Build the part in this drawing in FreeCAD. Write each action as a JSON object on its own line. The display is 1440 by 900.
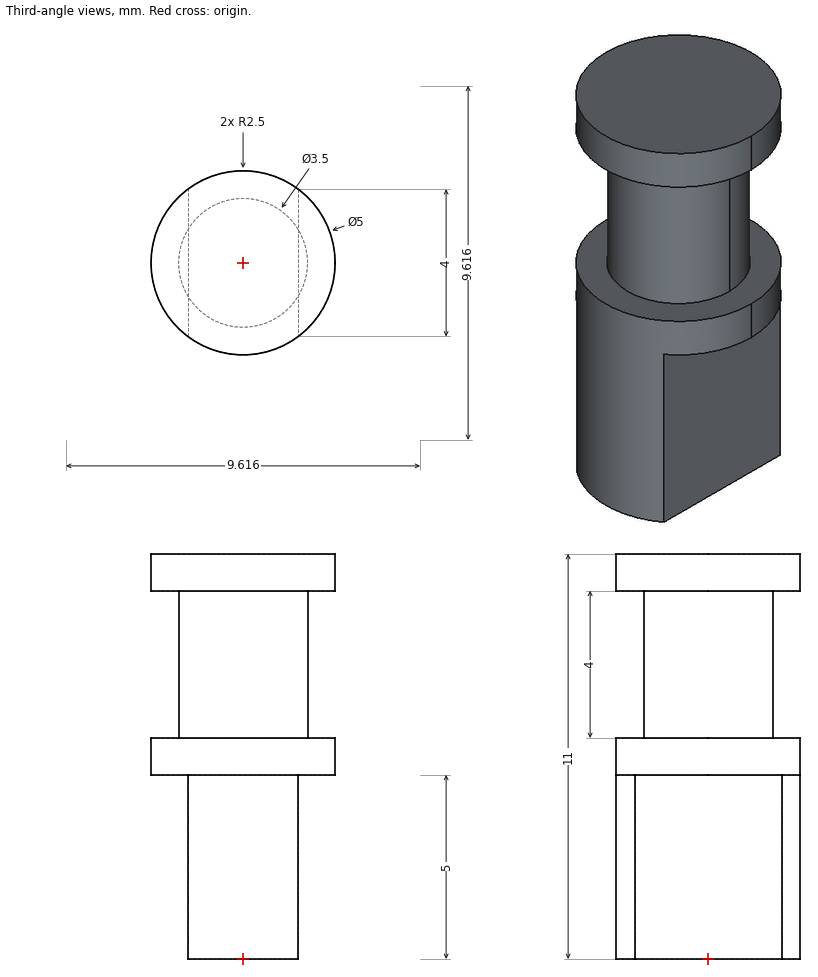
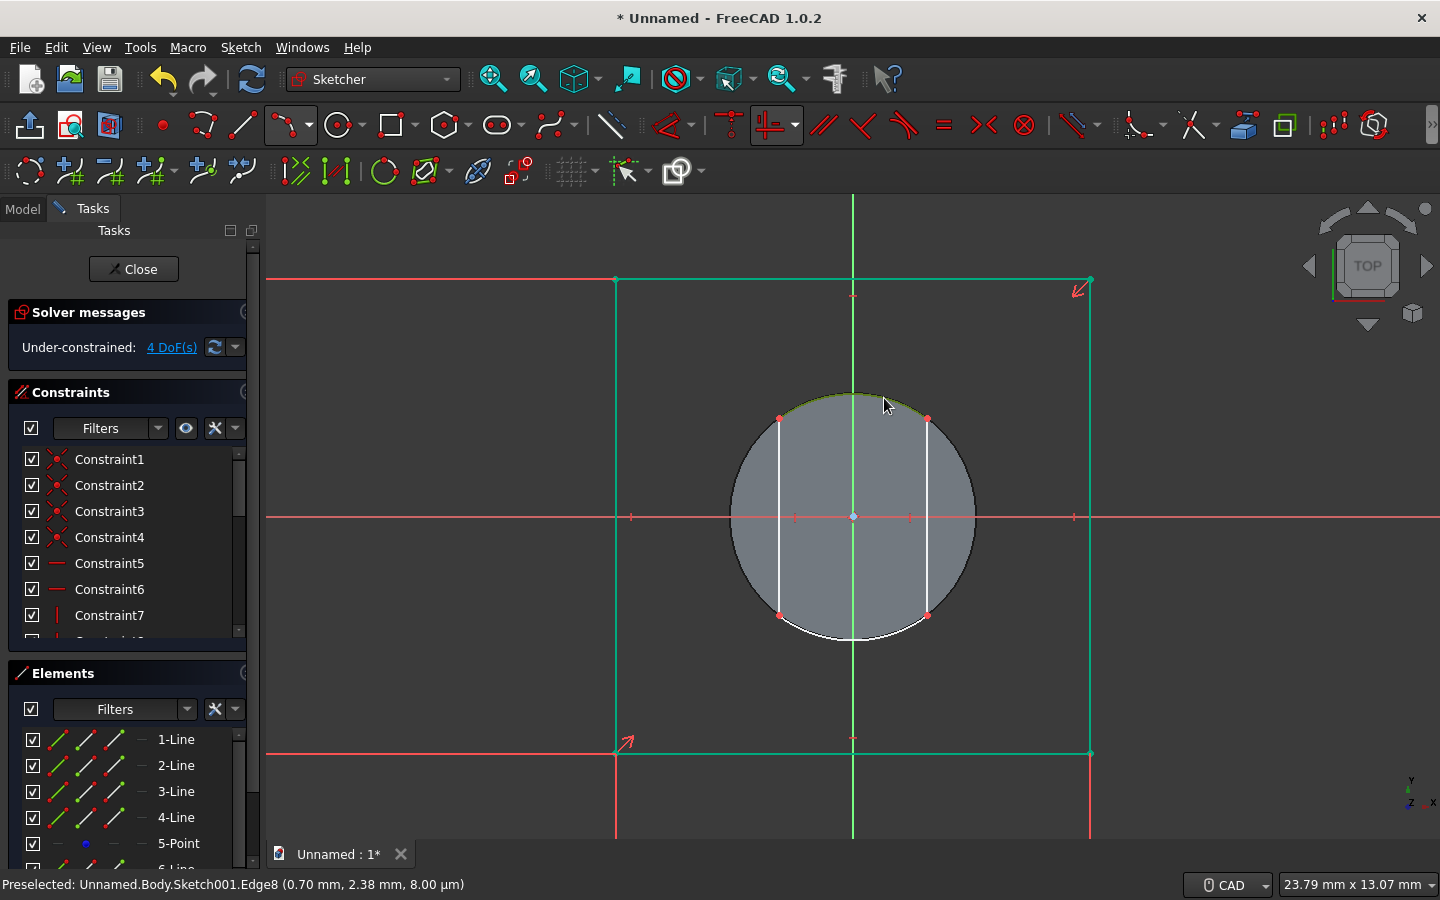
{"action": "left_click", "coordinate": [822, 636]}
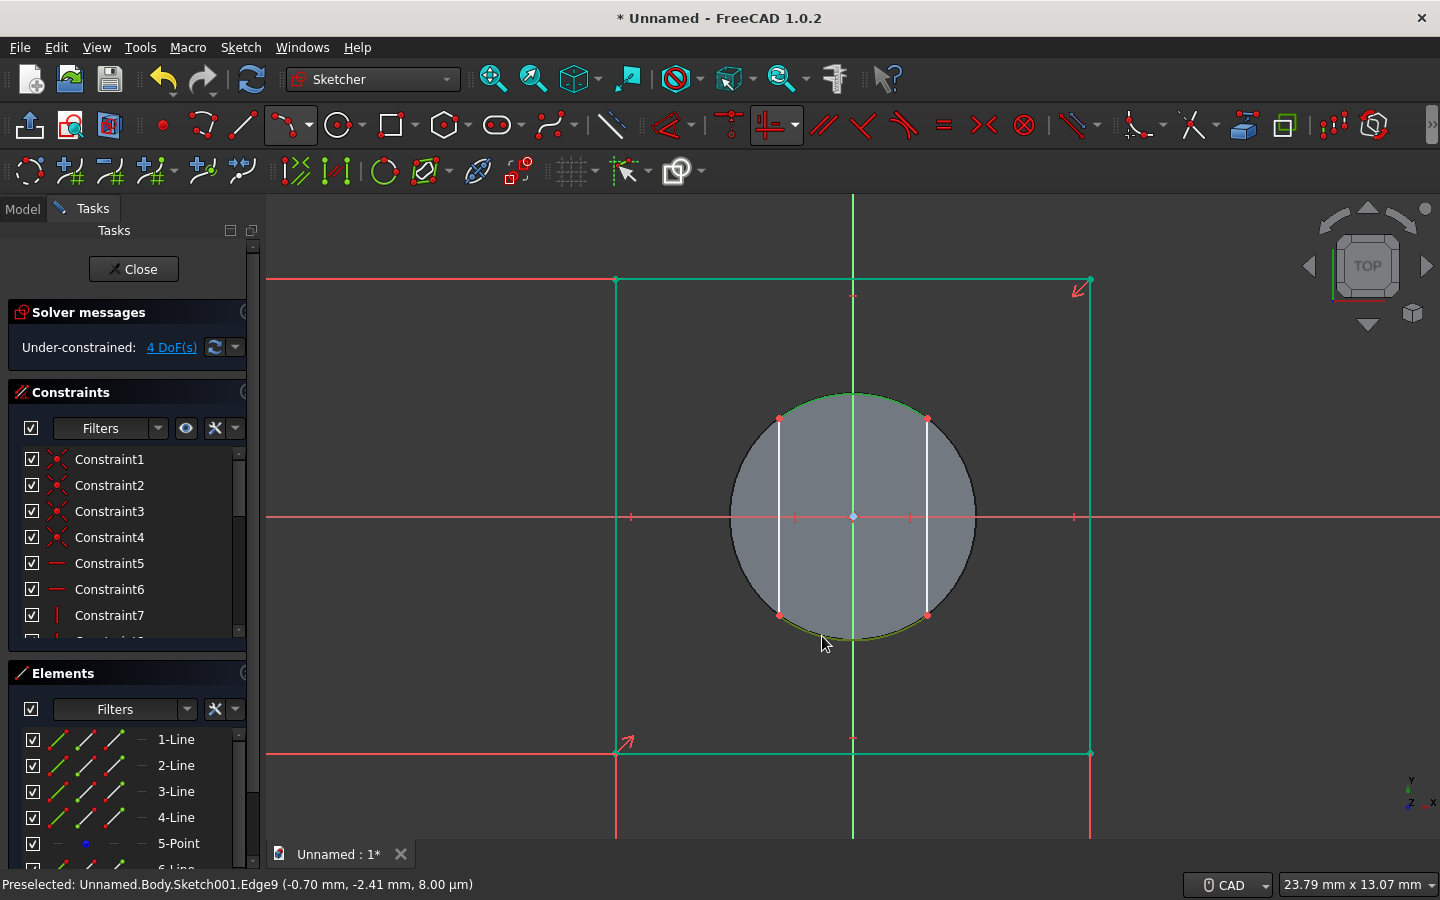
{"action": "key", "text": "e"}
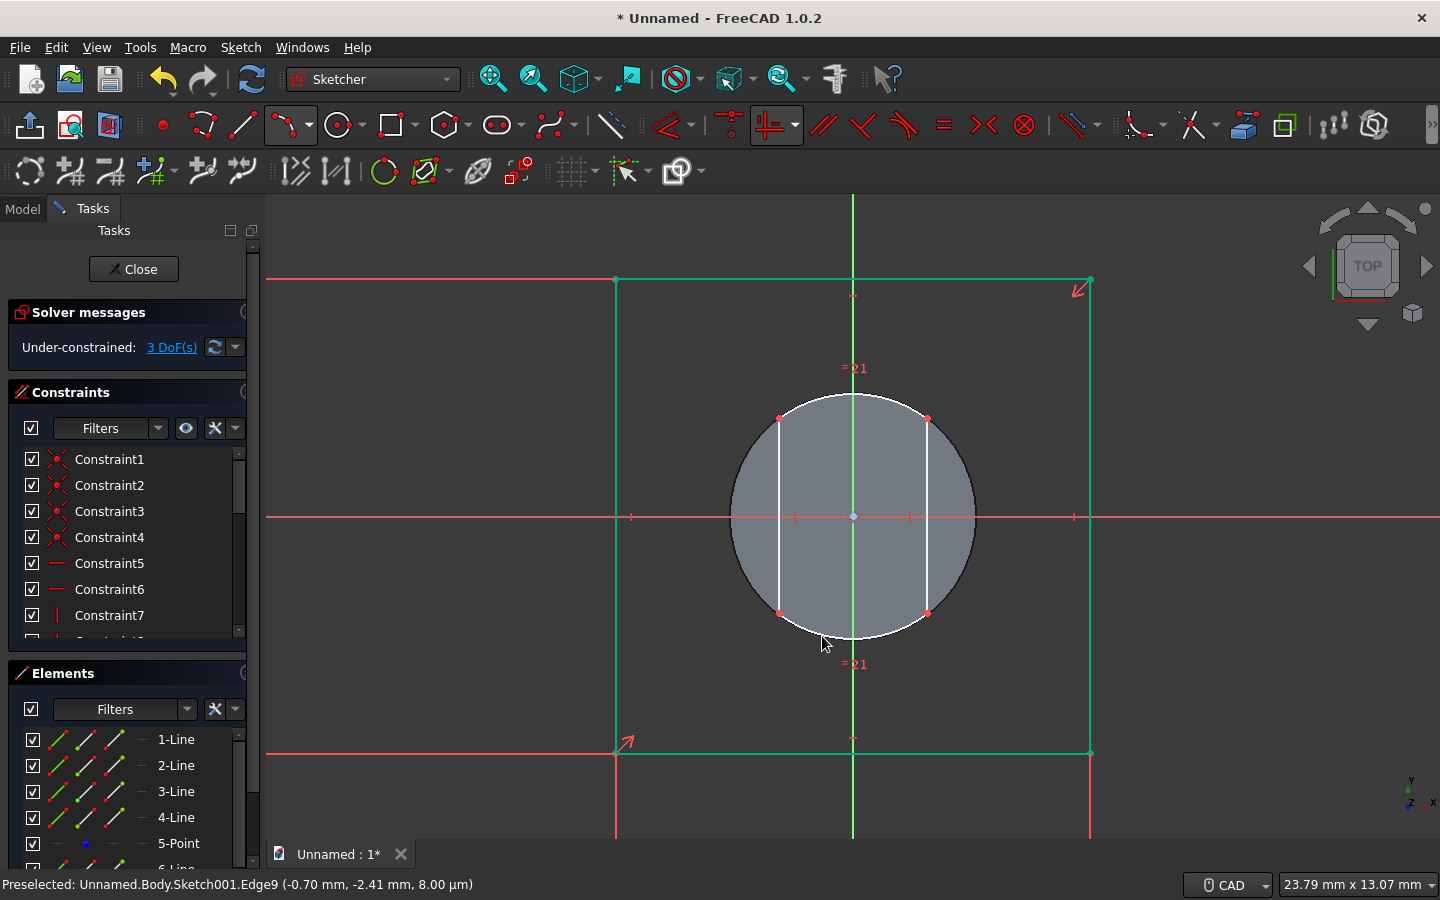
{"action": "left_click", "coordinate": [666, 126]}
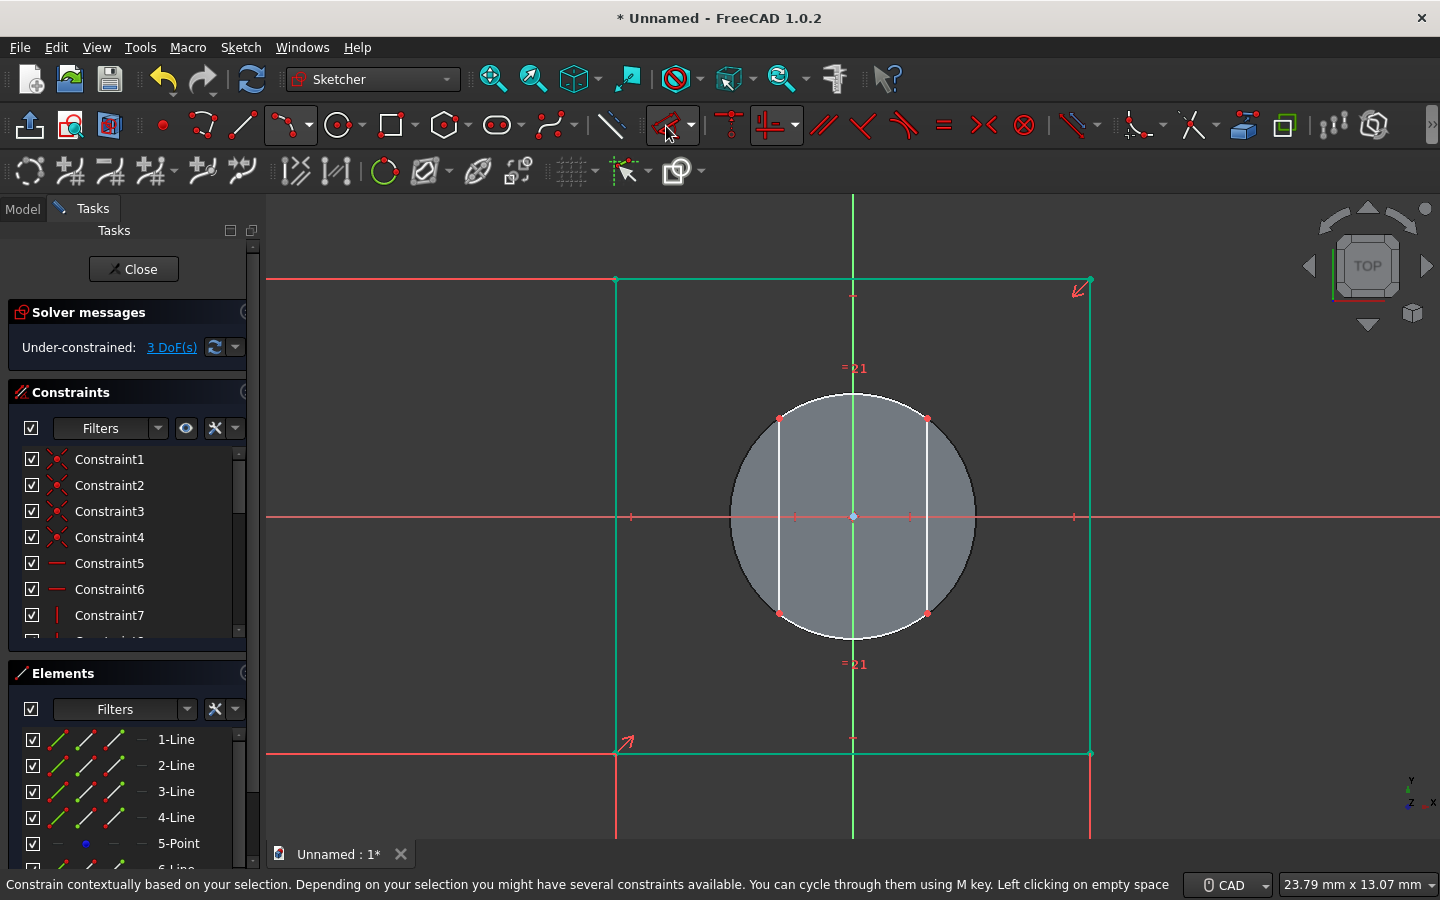
{"action": "left_click", "coordinate": [884, 398]}
{"action": "left_click", "coordinate": [892, 367]}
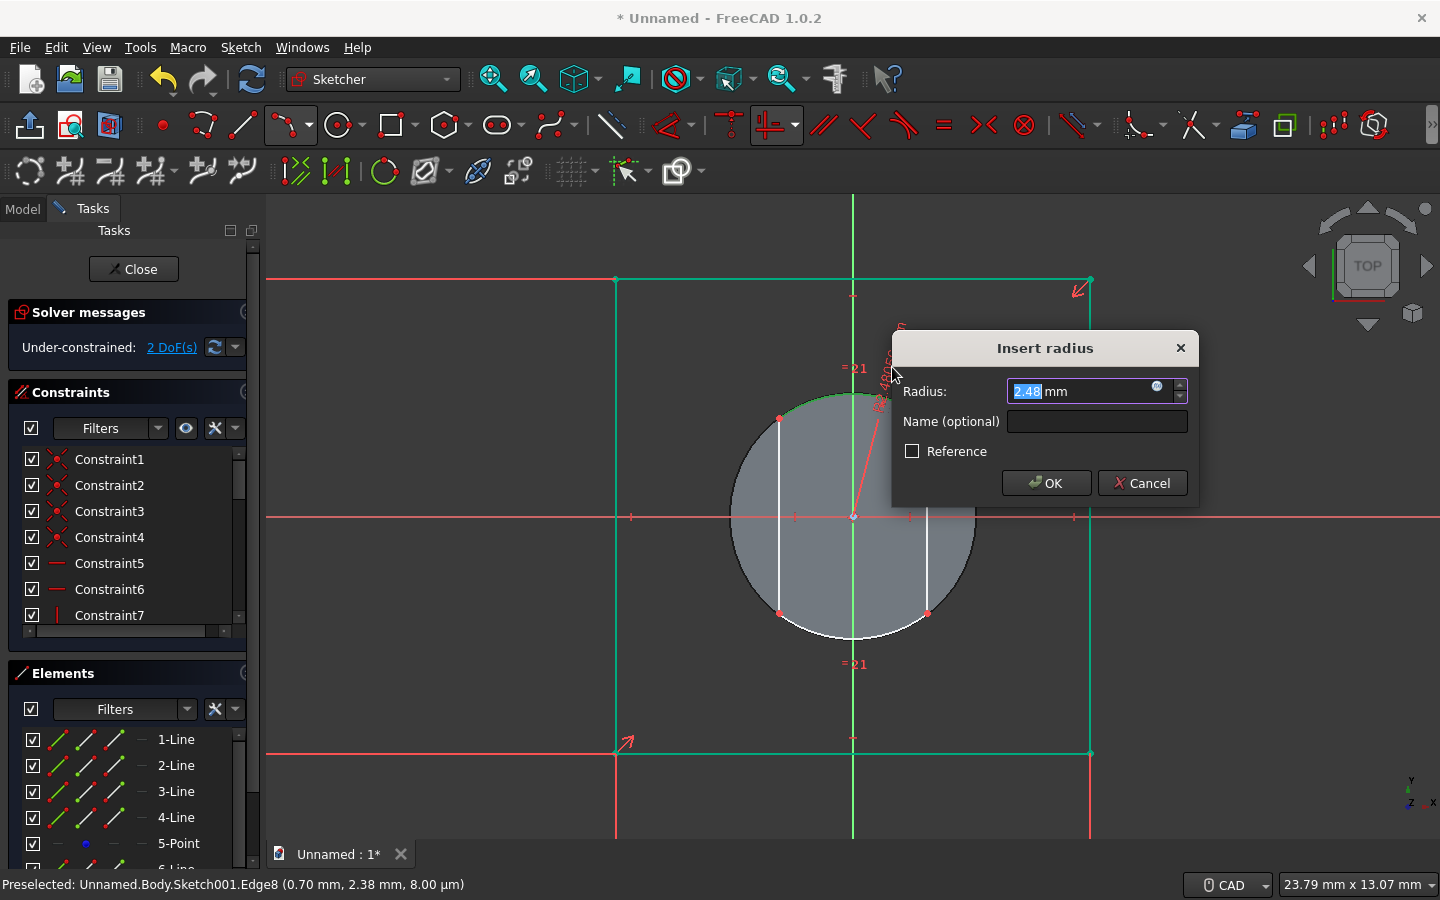
{"action": "type", "text": "2.5"}
{"action": "key", "text": "Return"}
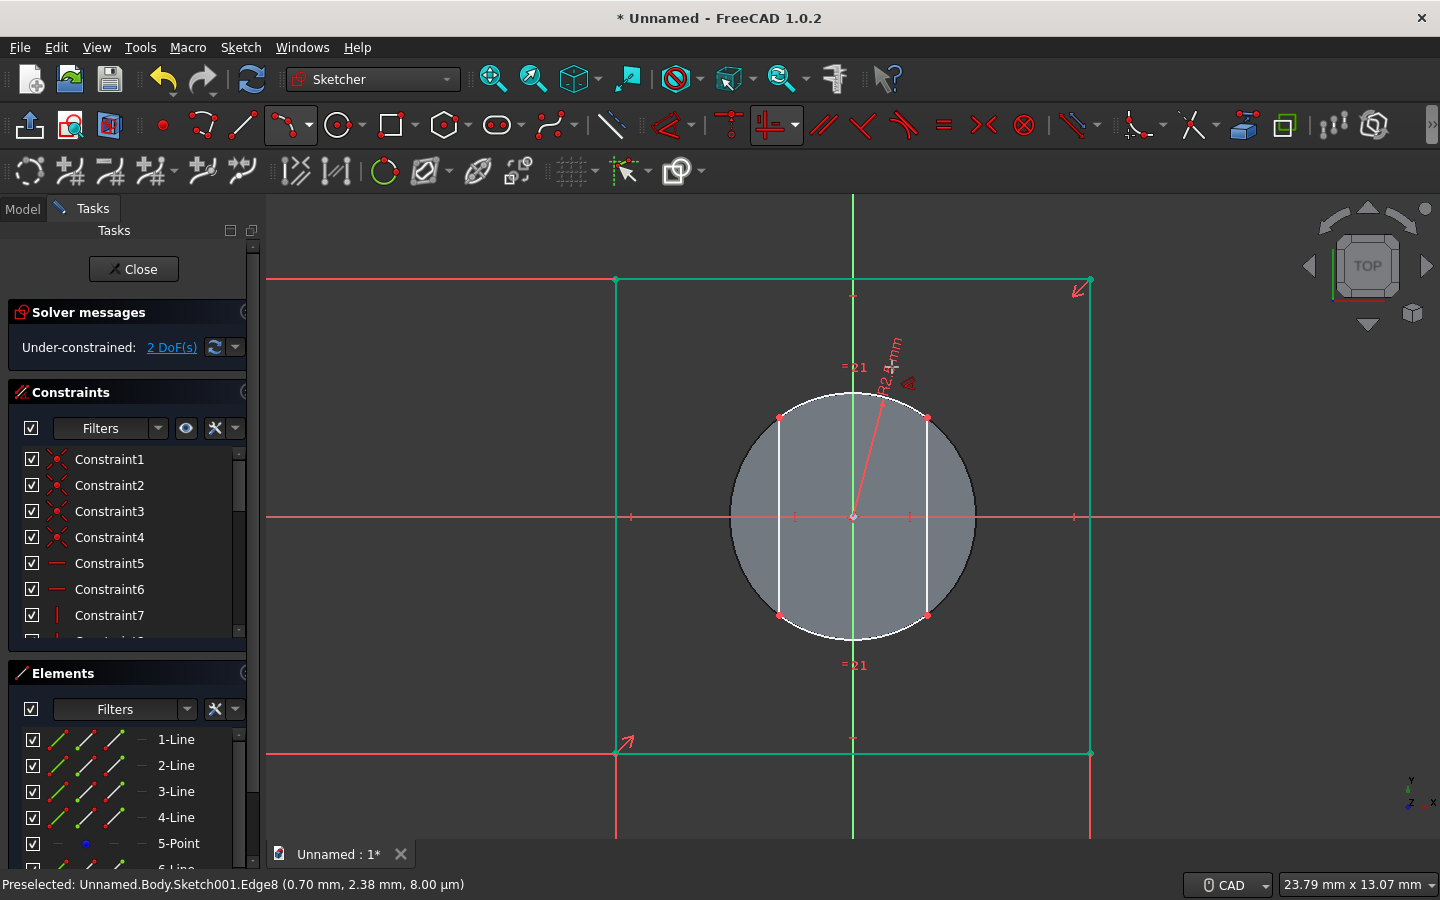
{"action": "left_click", "coordinate": [927, 556]}
{"action": "left_click", "coordinate": [961, 471]}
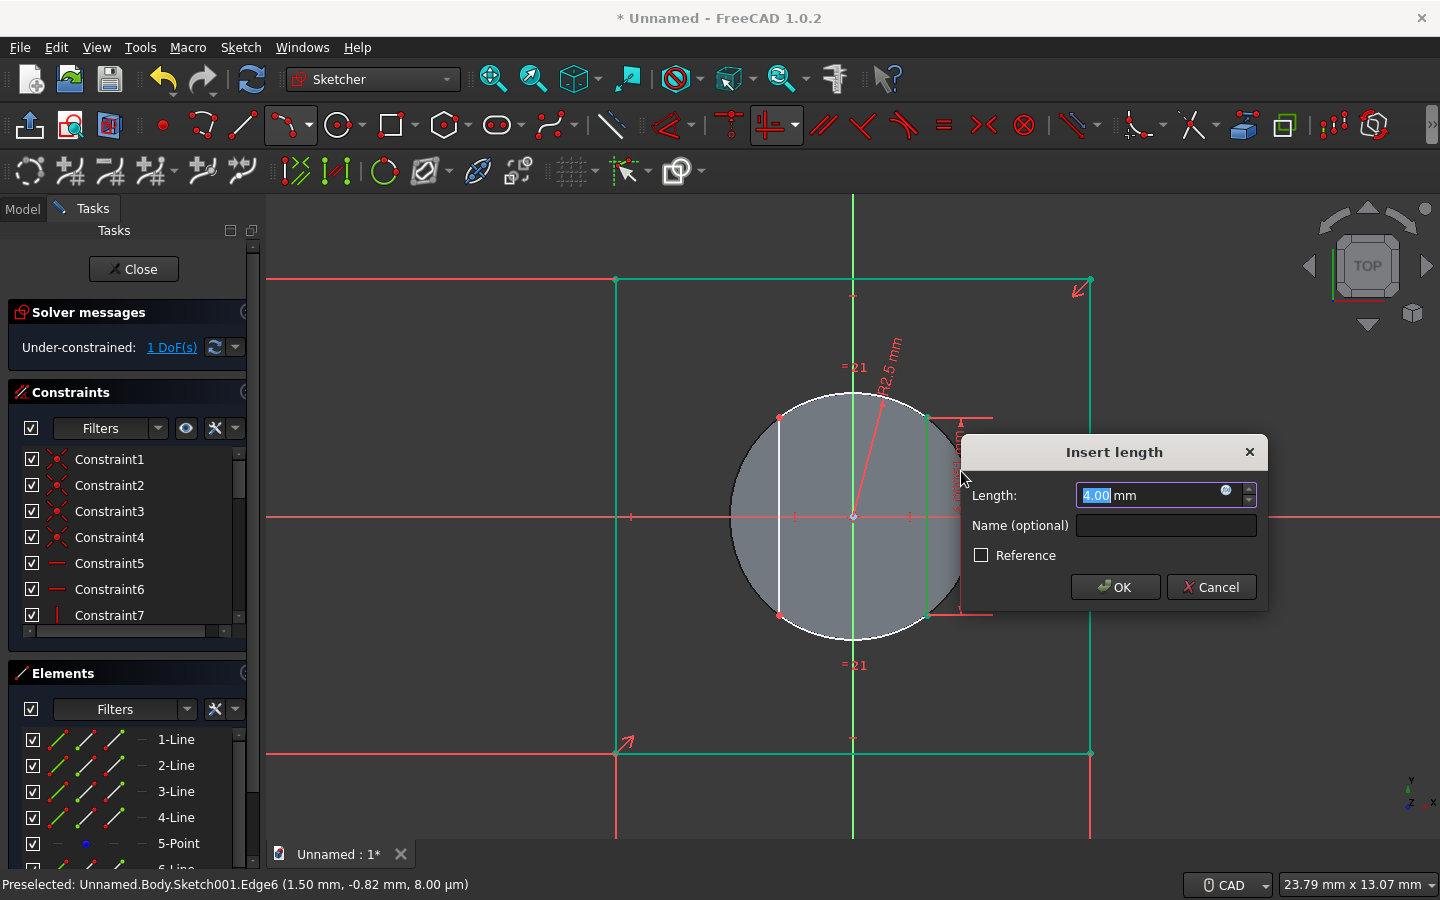
{"action": "type", "text": "4"}
{"action": "key", "text": "Return"}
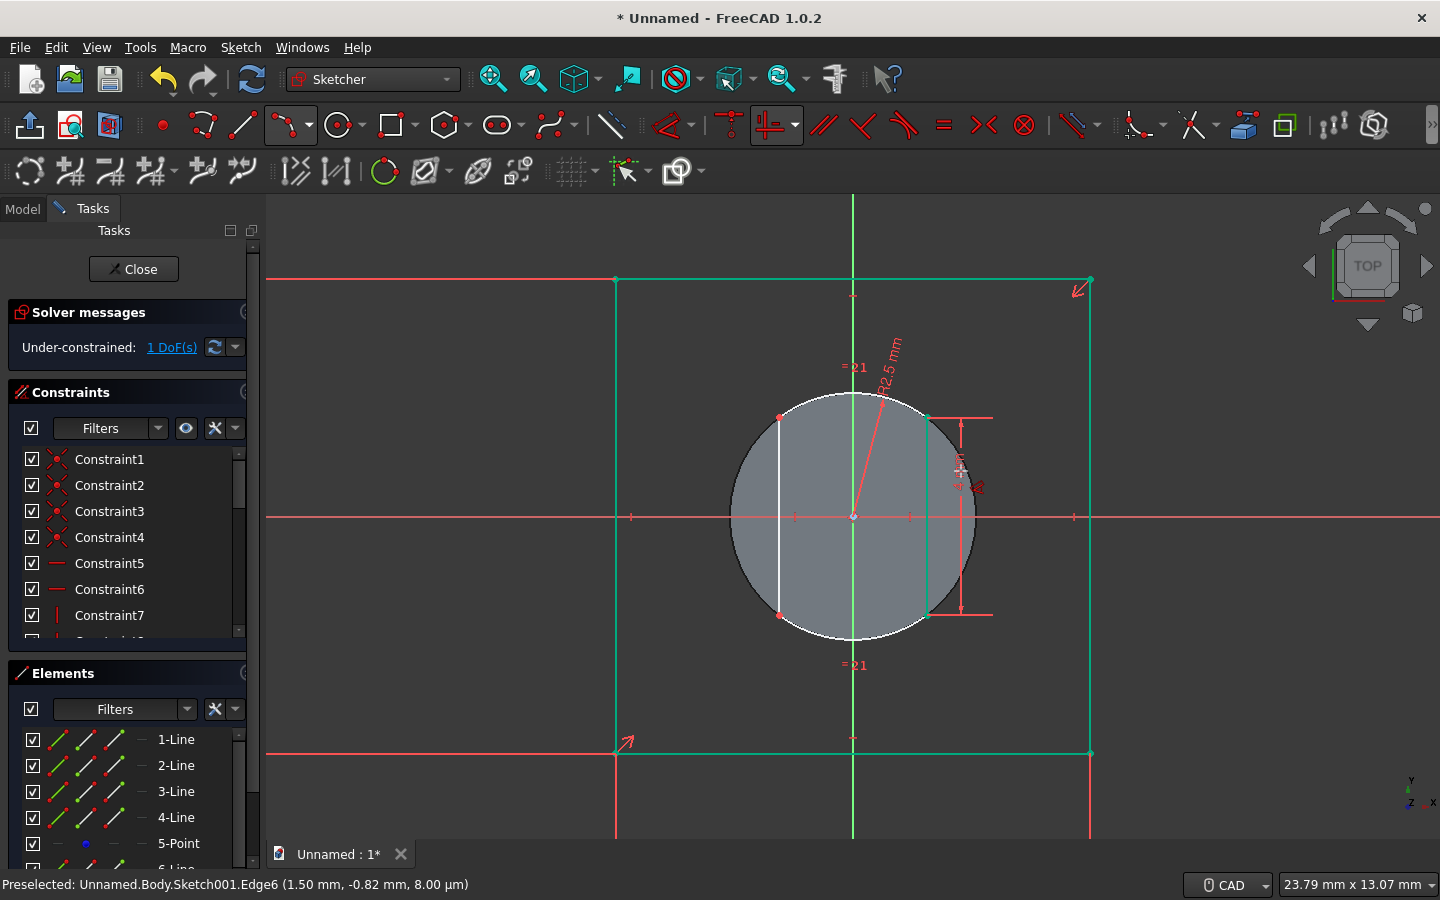
{"action": "left_click", "coordinate": [779, 477]}
{"action": "left_click", "coordinate": [745, 471]}